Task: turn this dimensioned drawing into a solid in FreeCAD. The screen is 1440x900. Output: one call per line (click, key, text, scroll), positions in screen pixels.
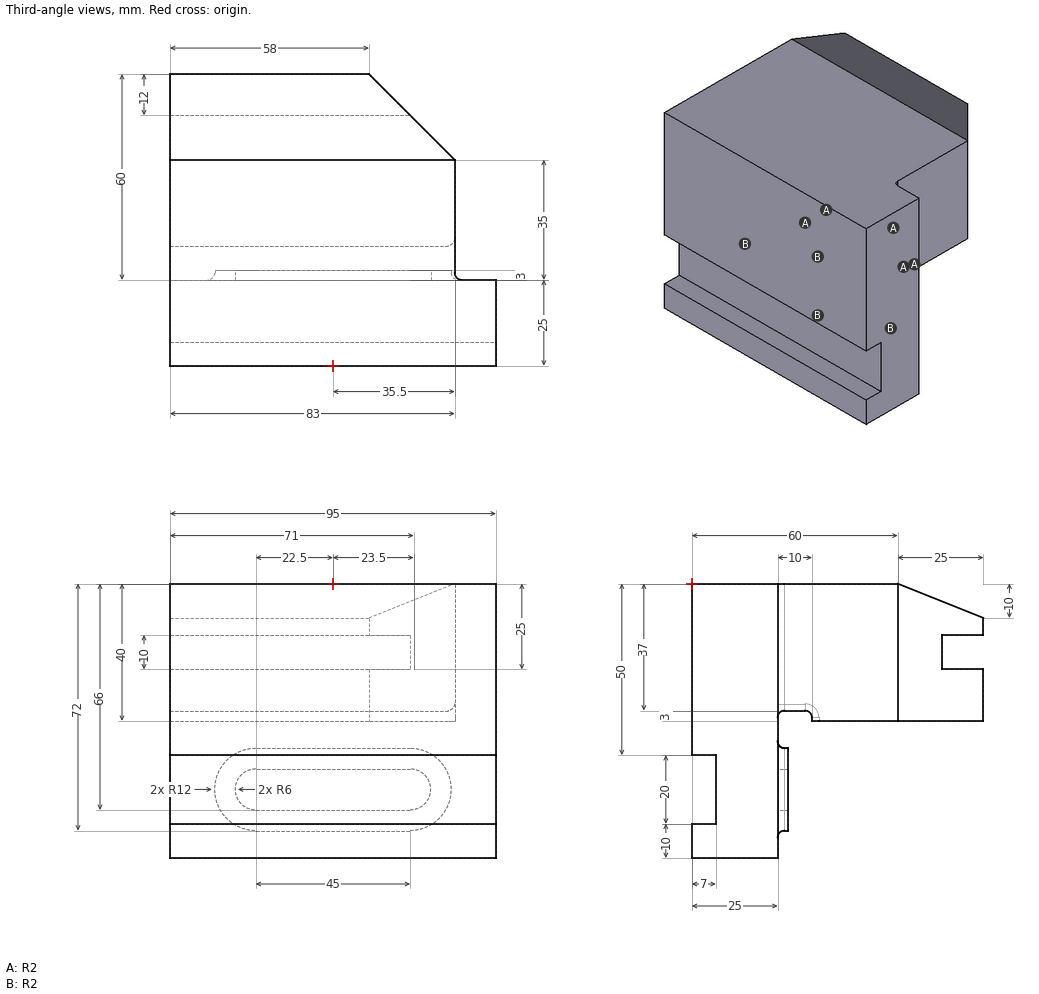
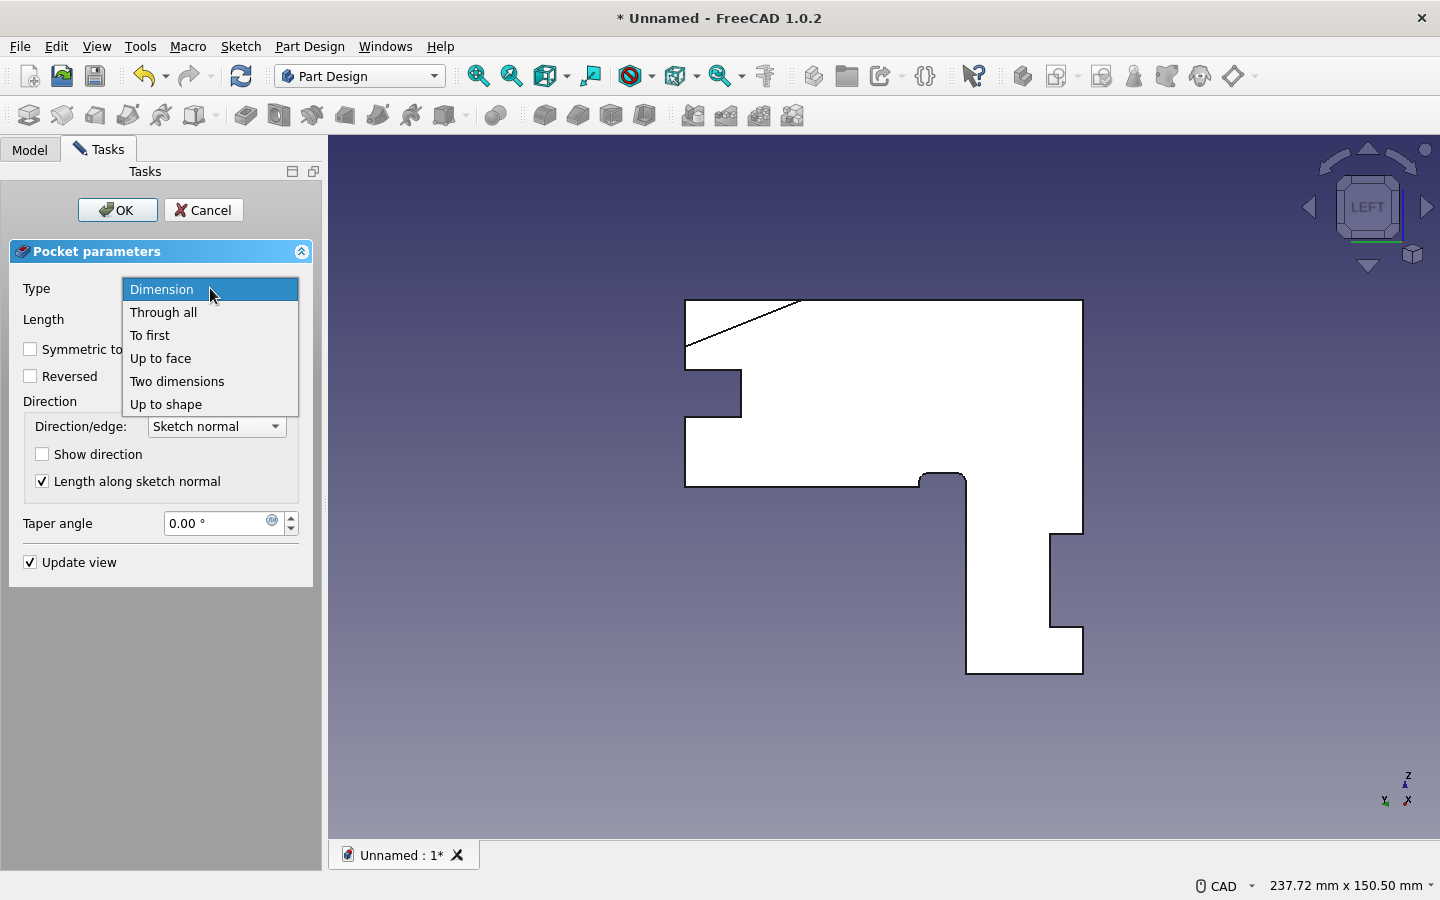
click(208, 312)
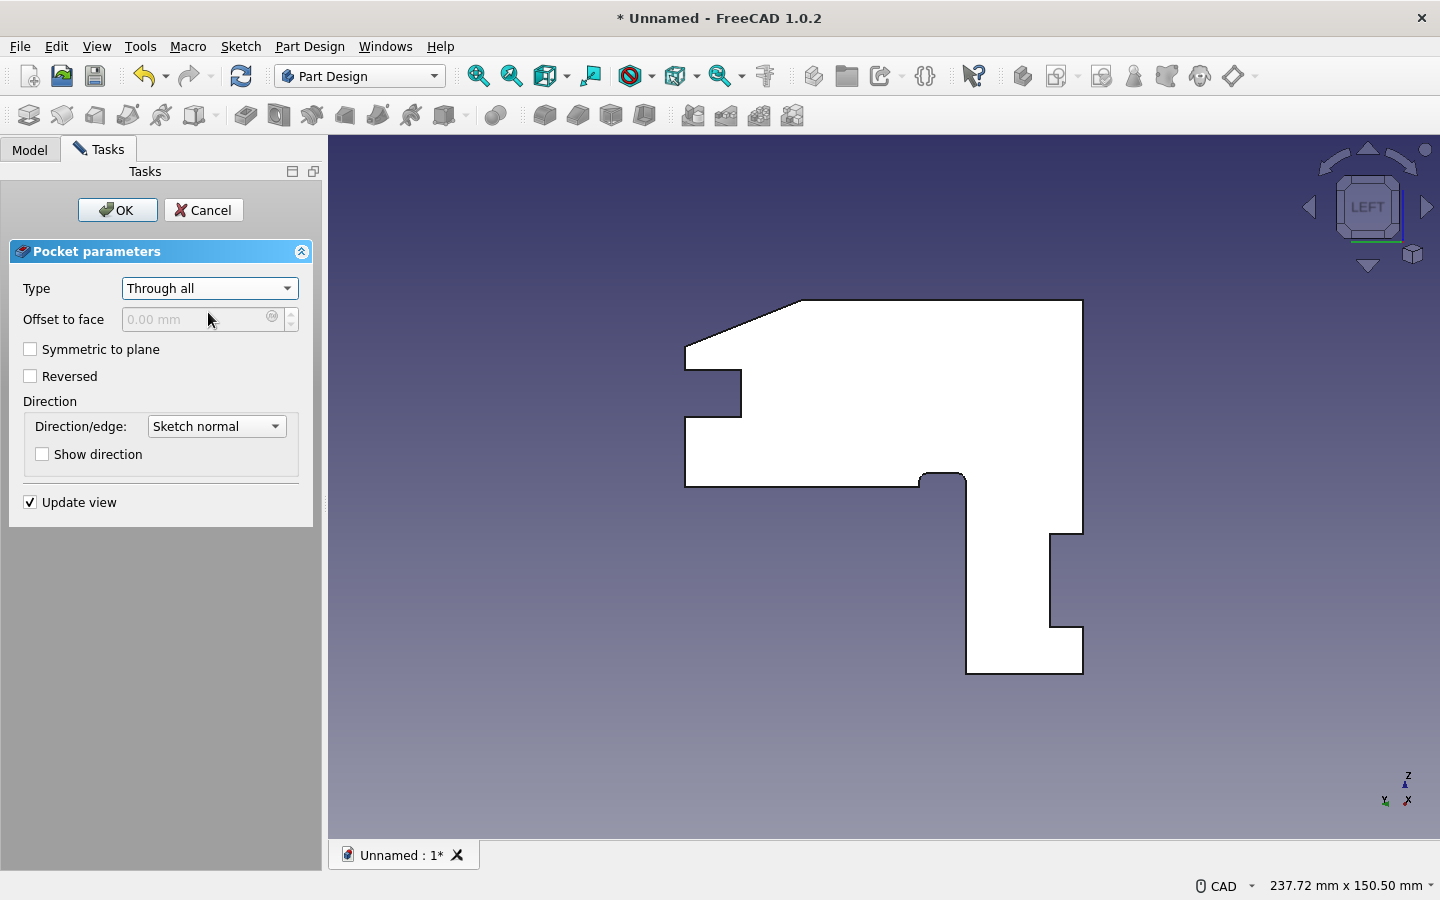
click(118, 210)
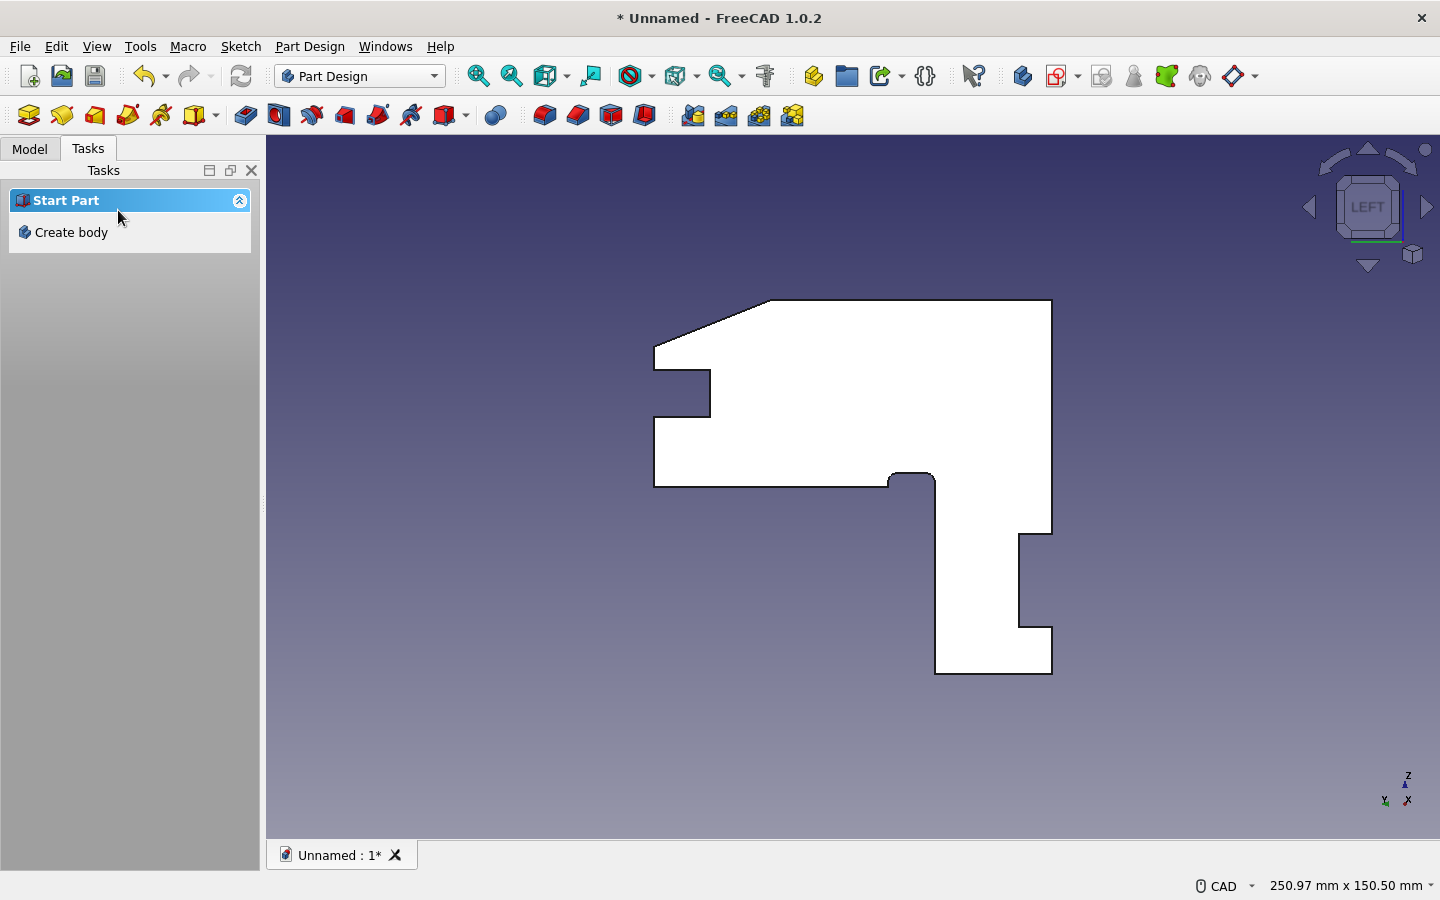
key(4)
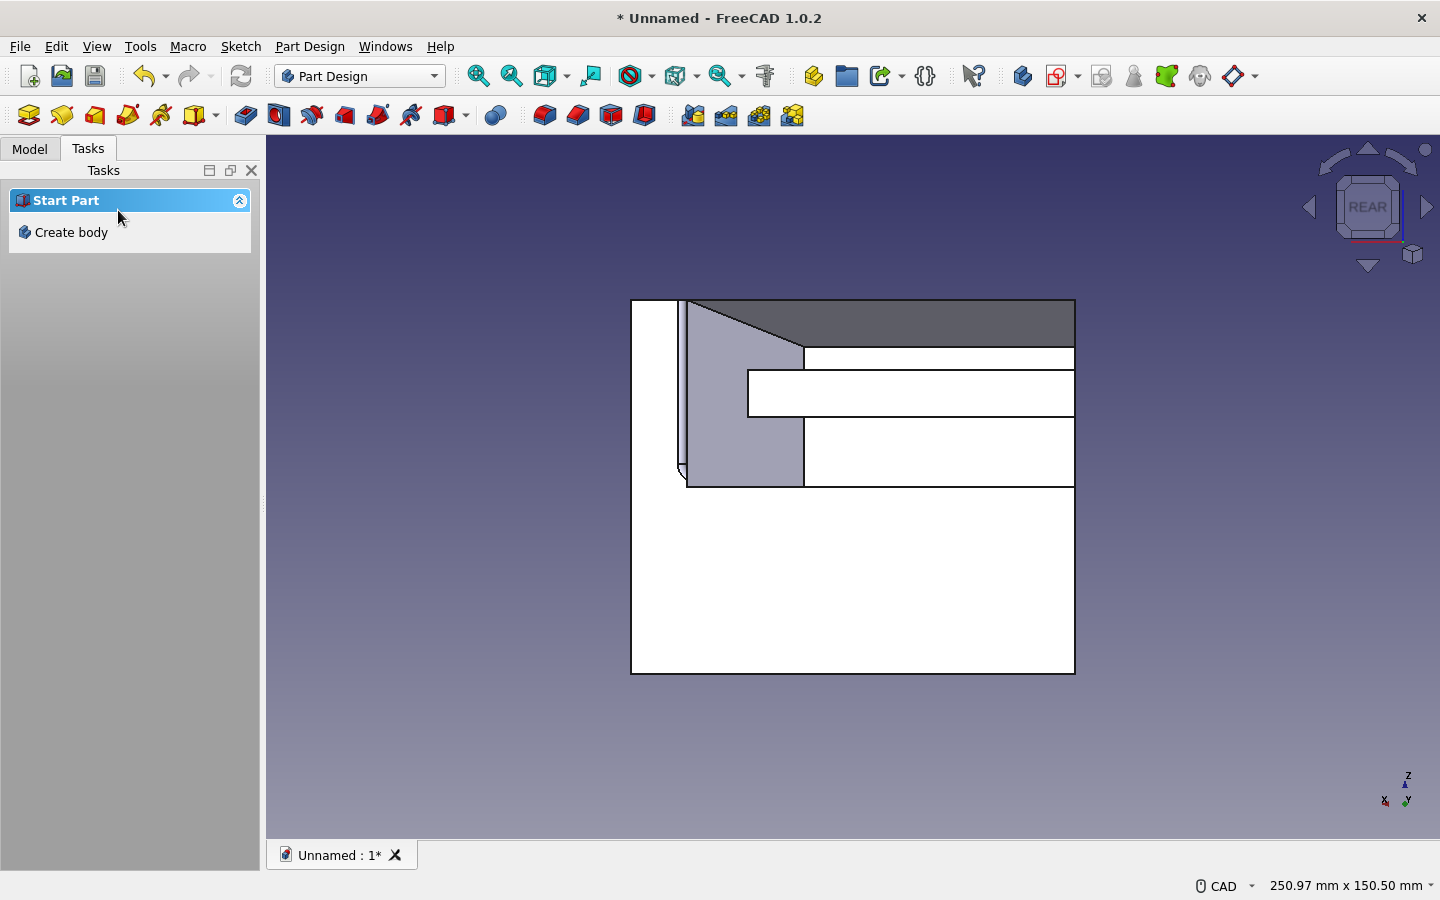
click(790, 593)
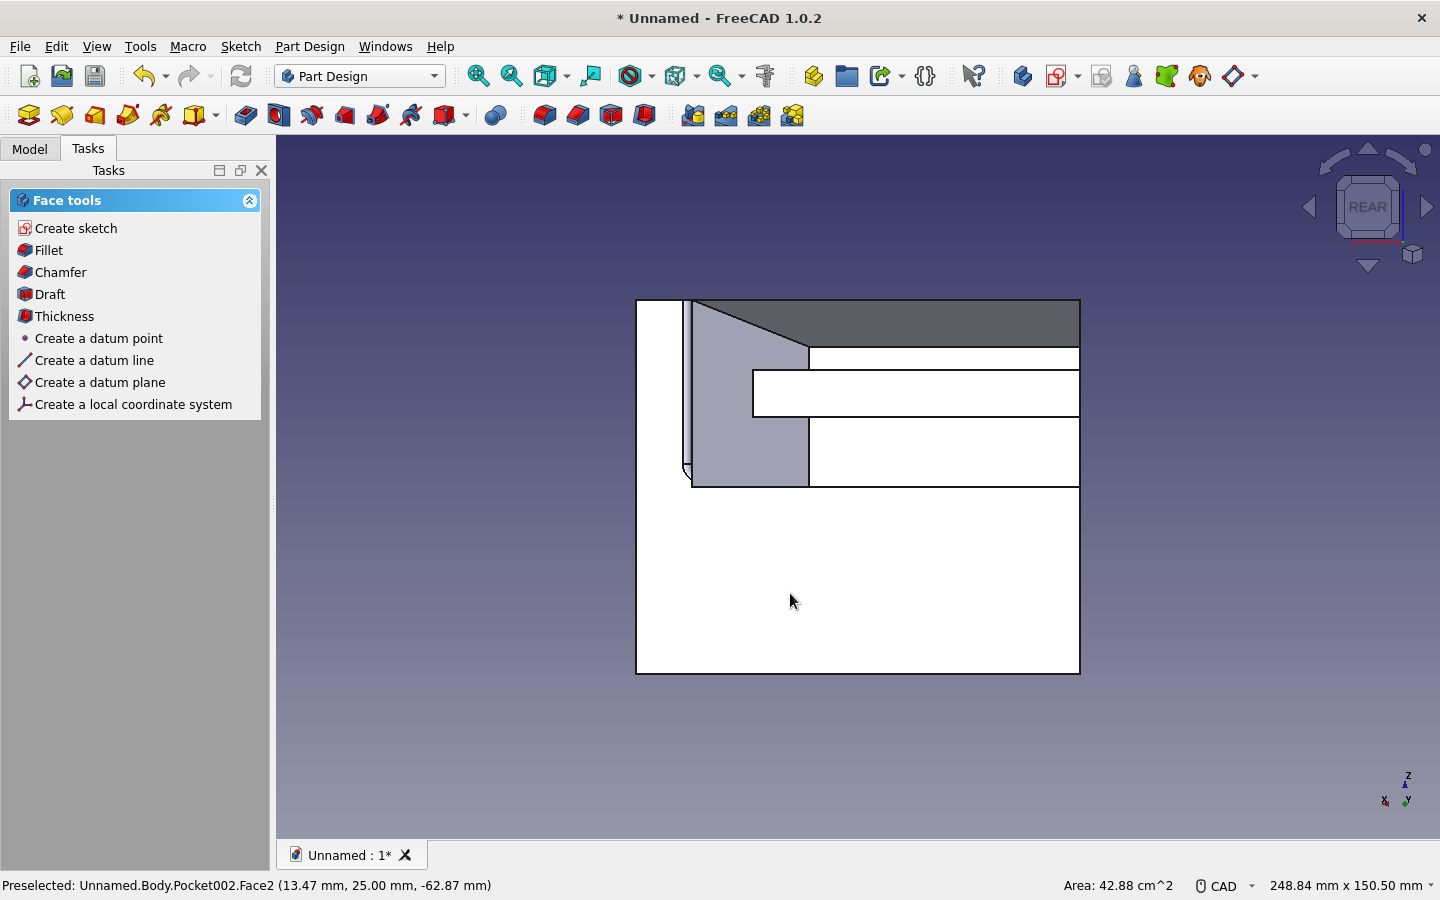
click(1056, 76)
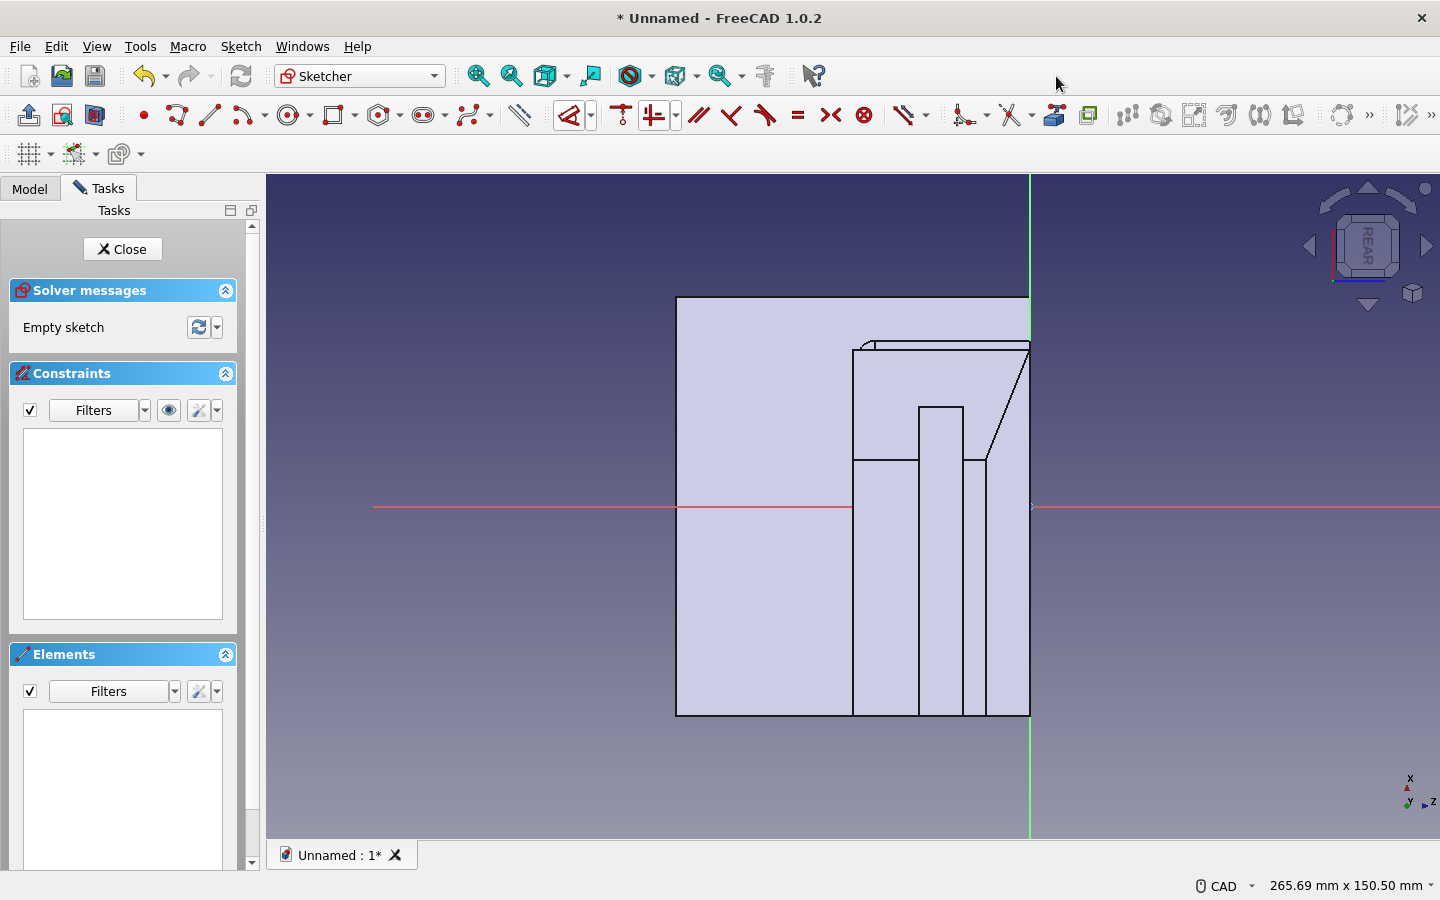
scroll(1046, 507, up, 2)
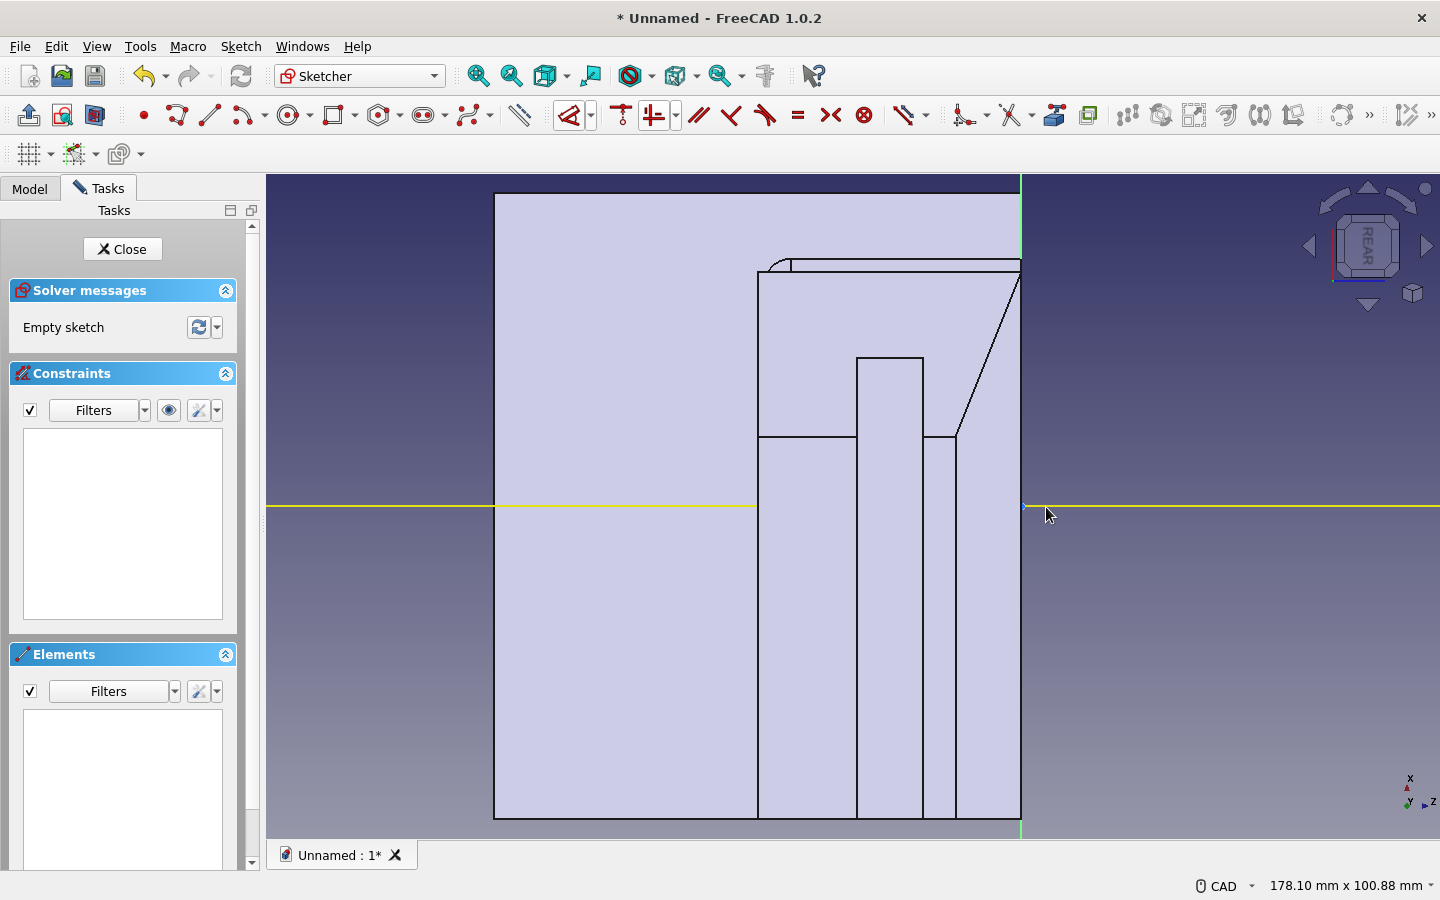
click(422, 116)